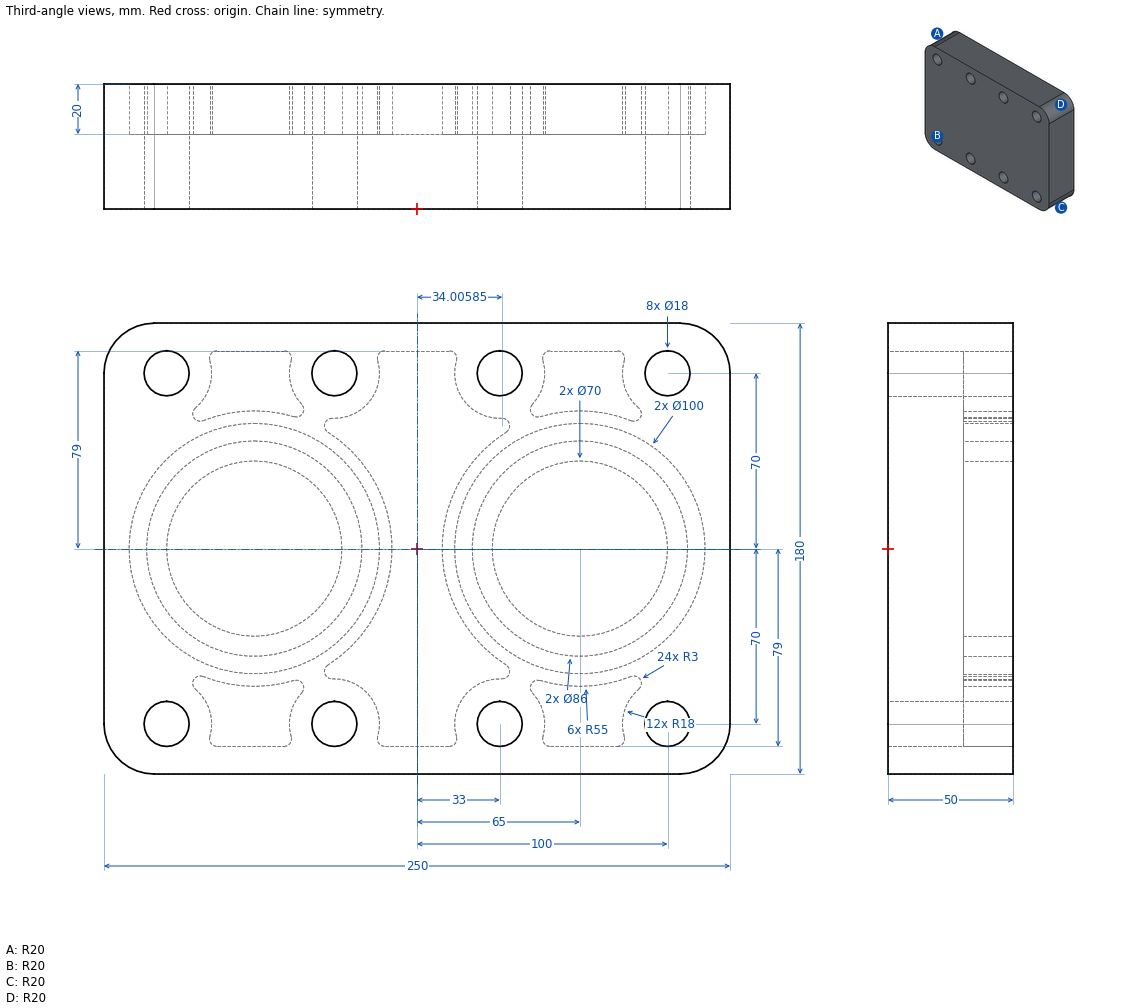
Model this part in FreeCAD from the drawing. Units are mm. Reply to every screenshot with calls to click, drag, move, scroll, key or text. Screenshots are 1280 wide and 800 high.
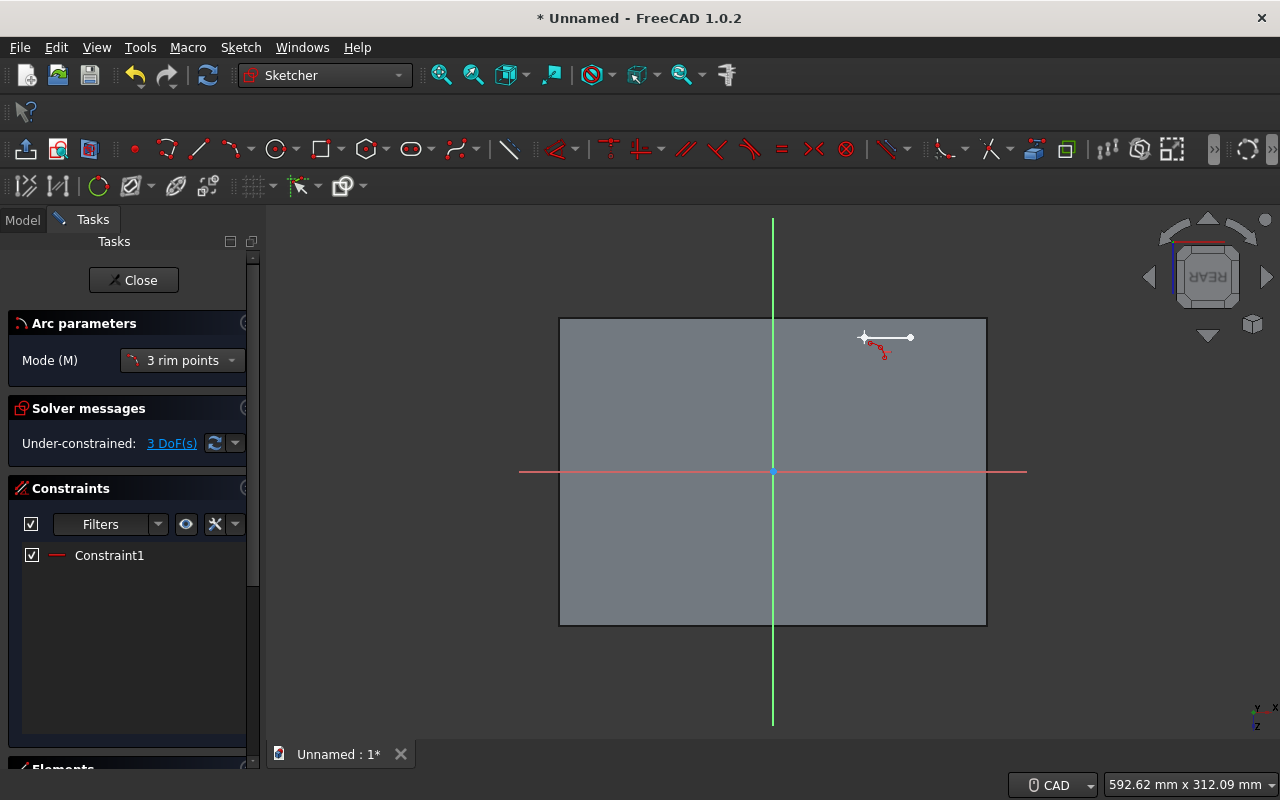
click(864, 338)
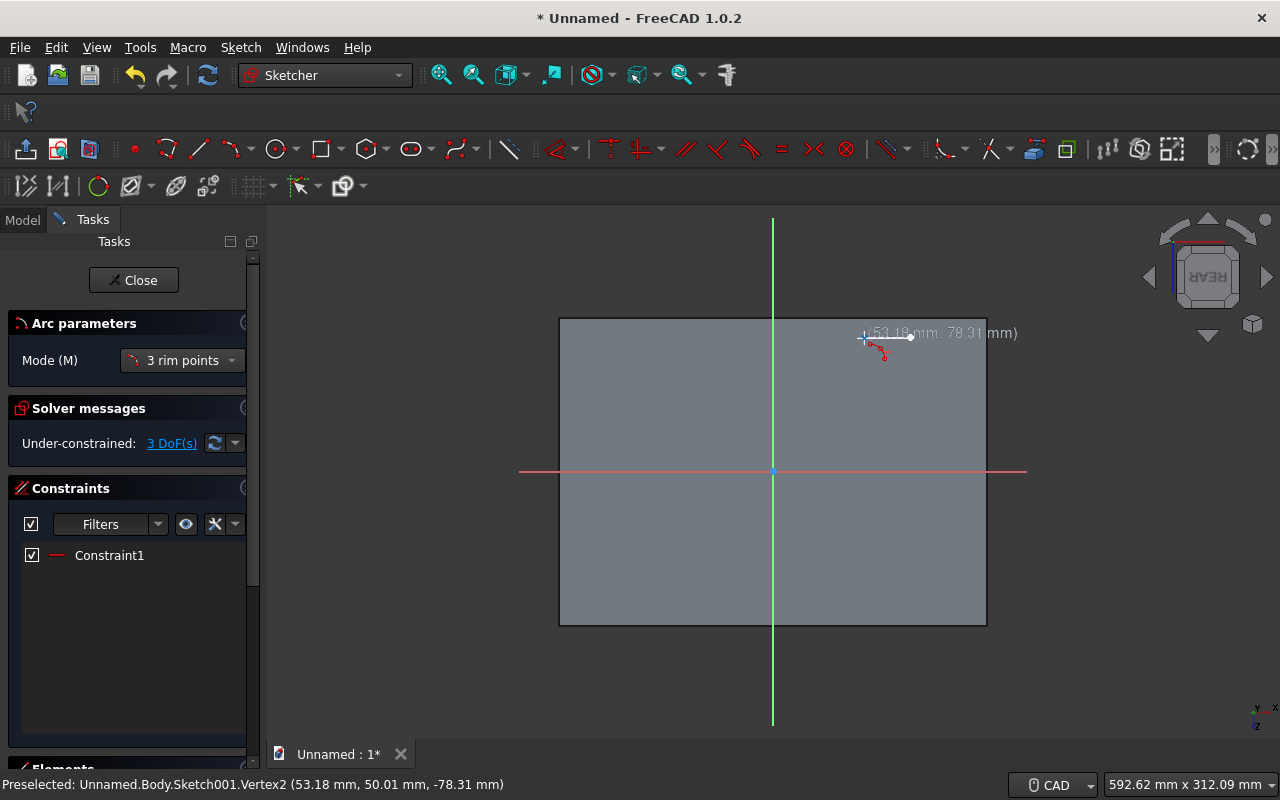
scroll(859, 343, up, 4)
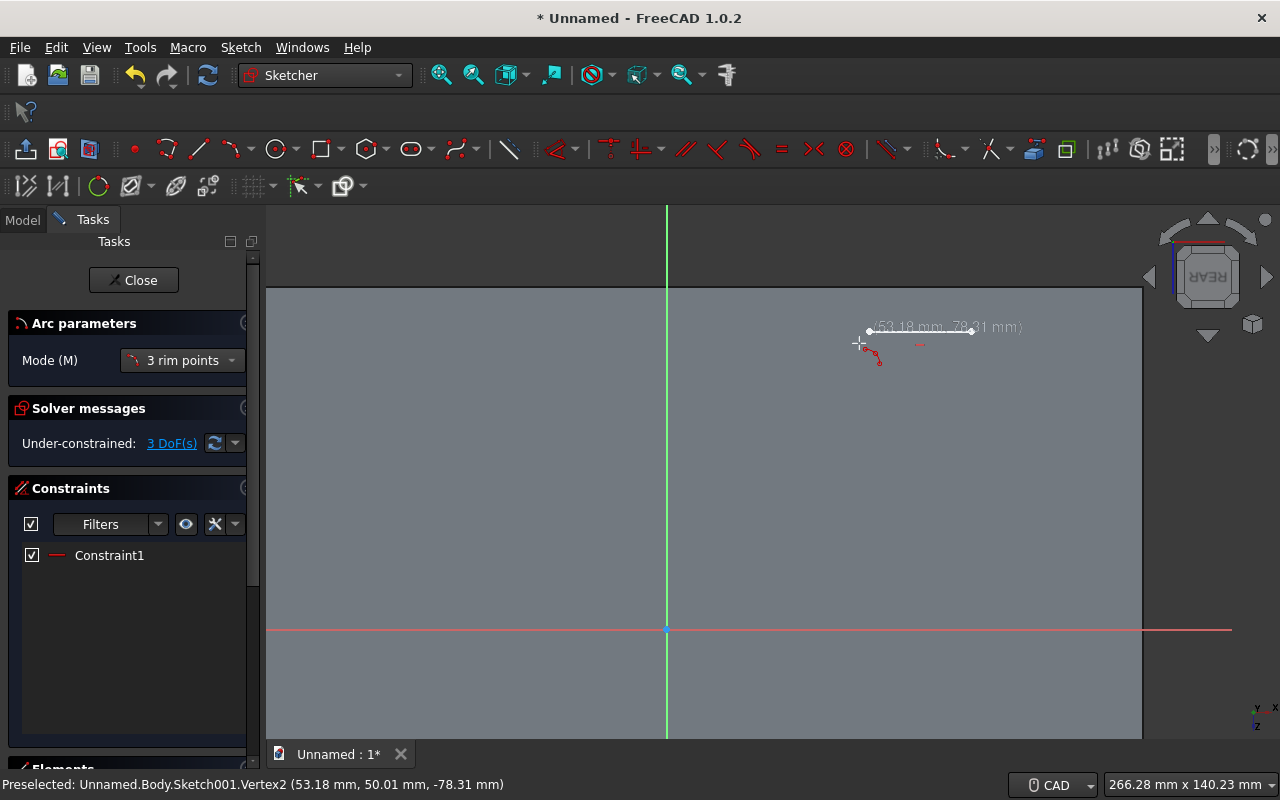
click(858, 344)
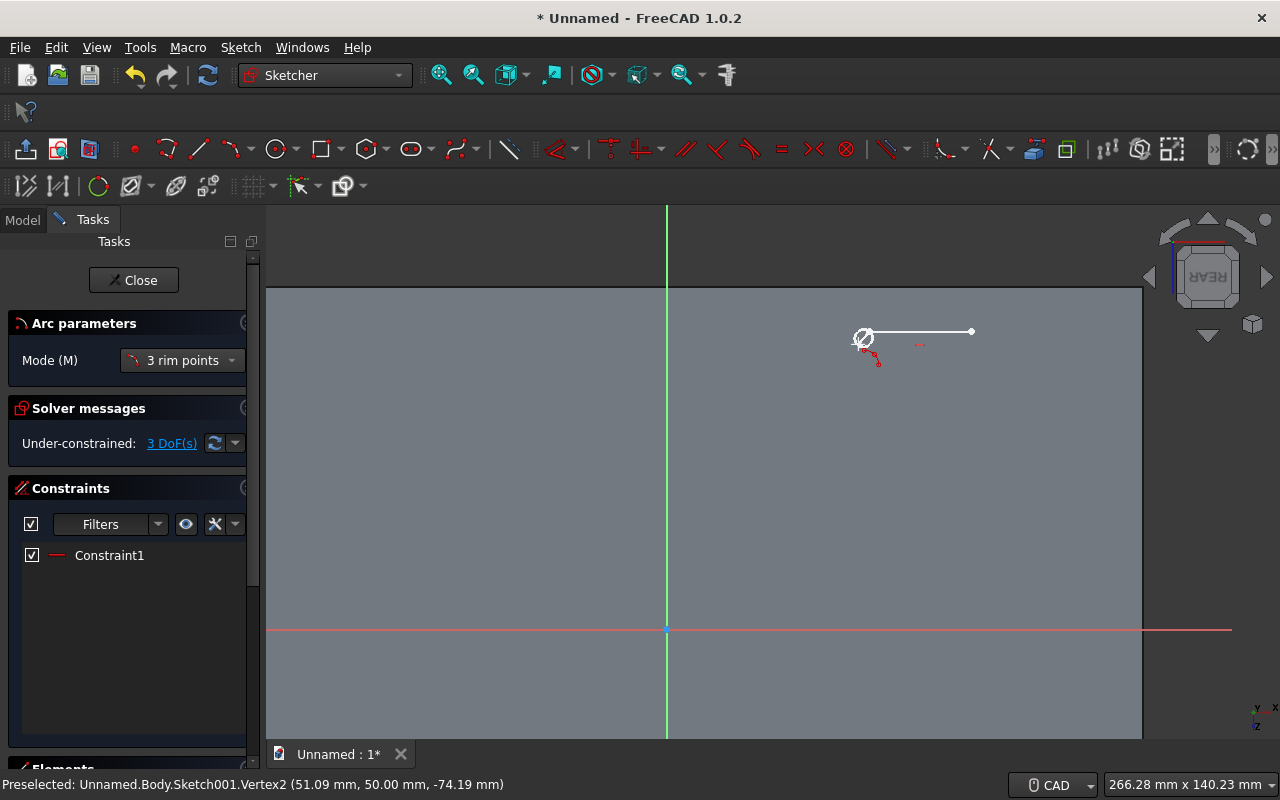
scroll(860, 334, up, 7)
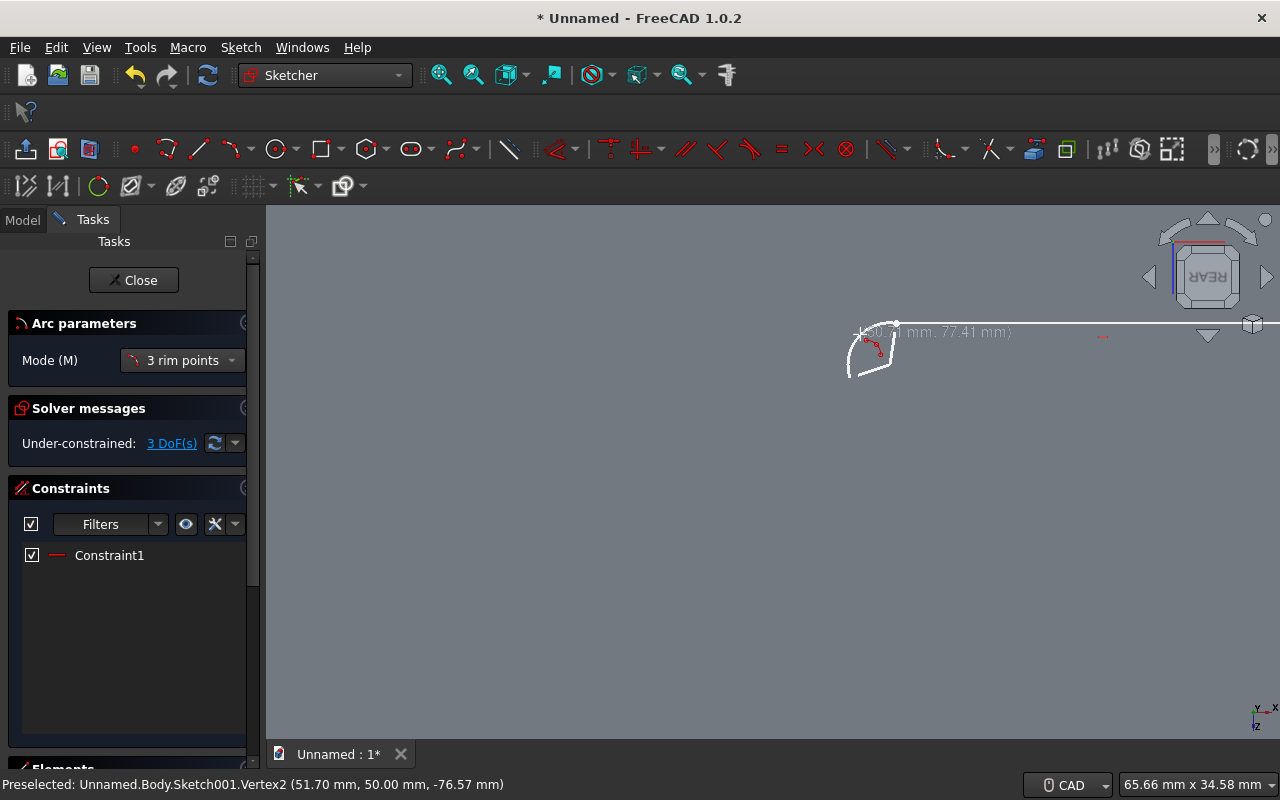
click(858, 331)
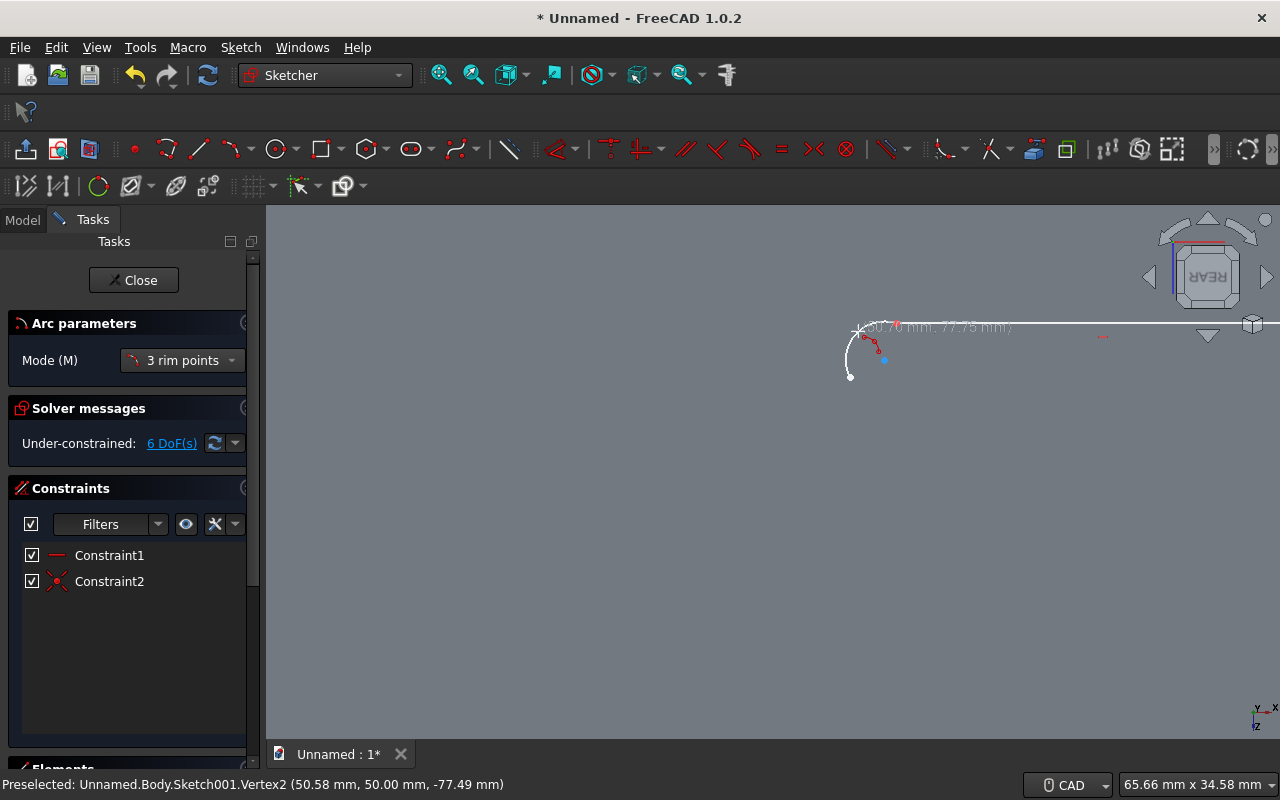
scroll(803, 306, down, 10)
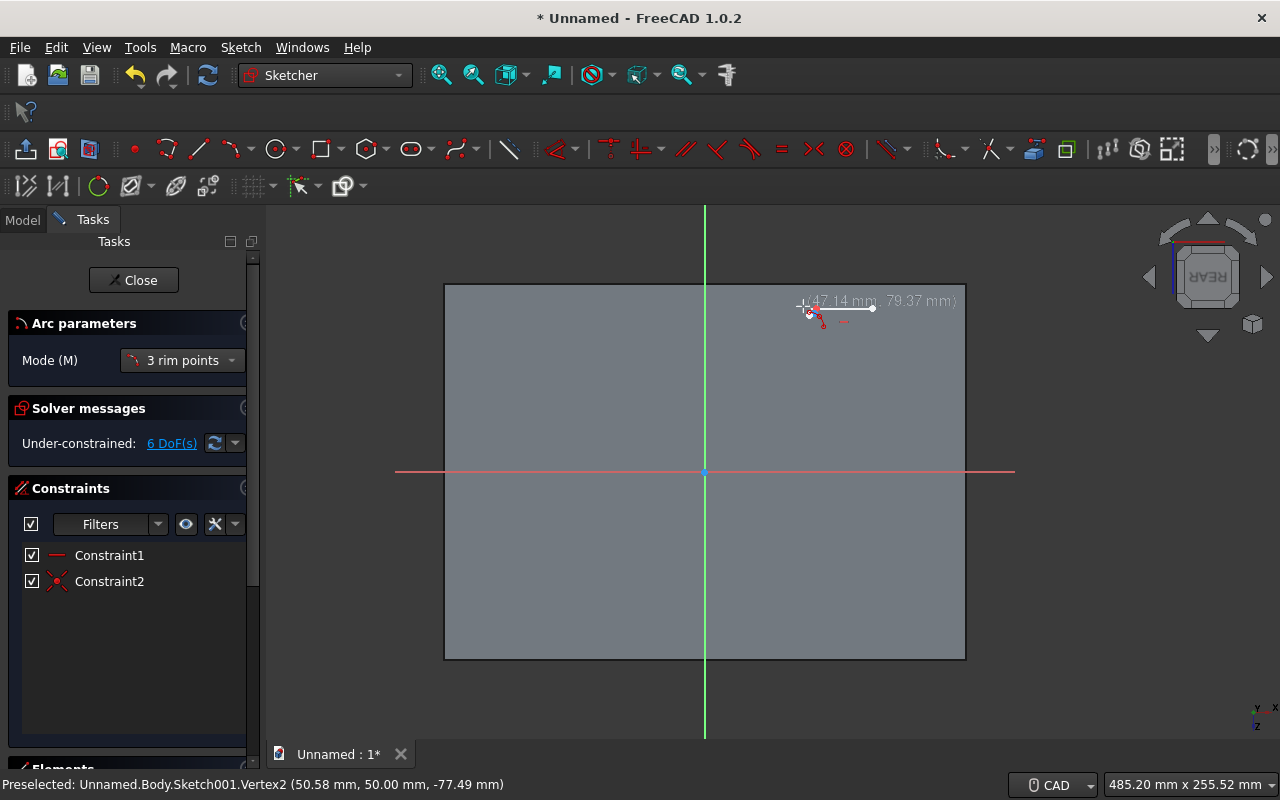
scroll(810, 315, up, 5)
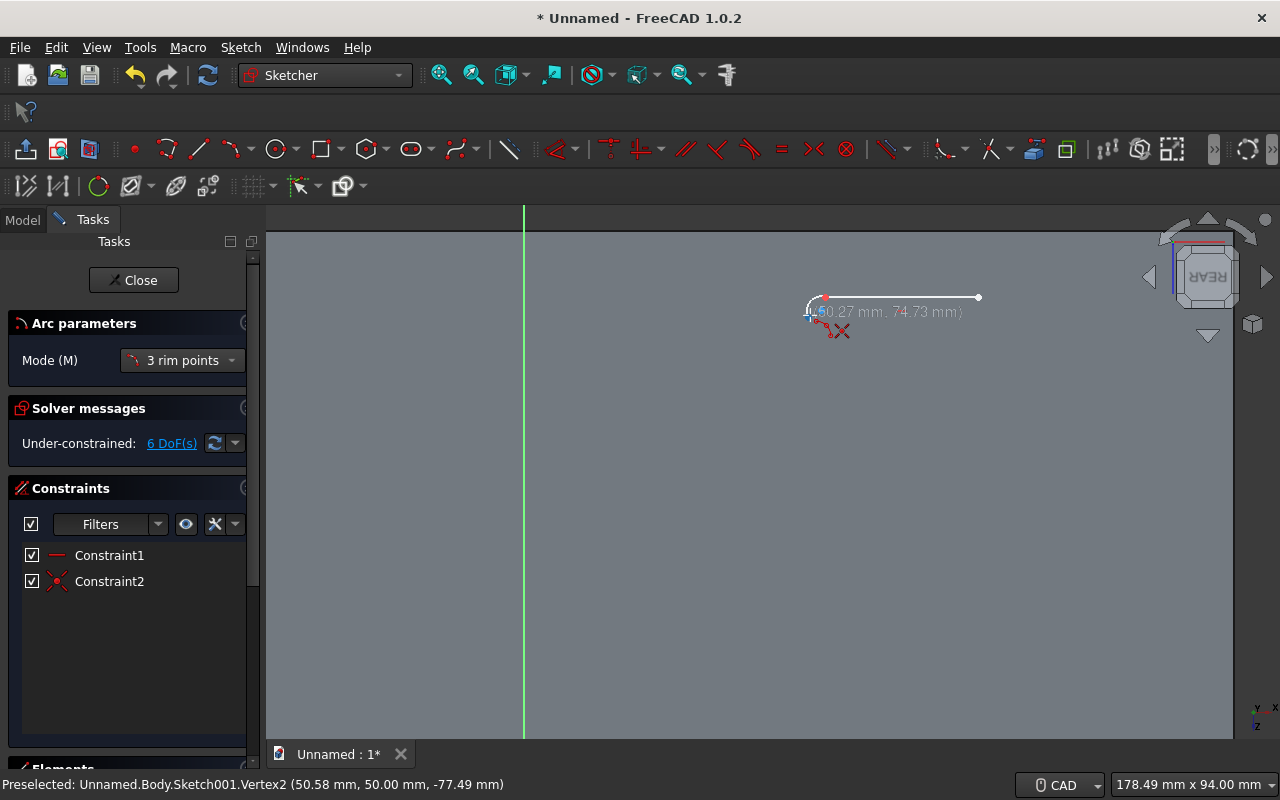
click(809, 317)
click(785, 415)
click(810, 368)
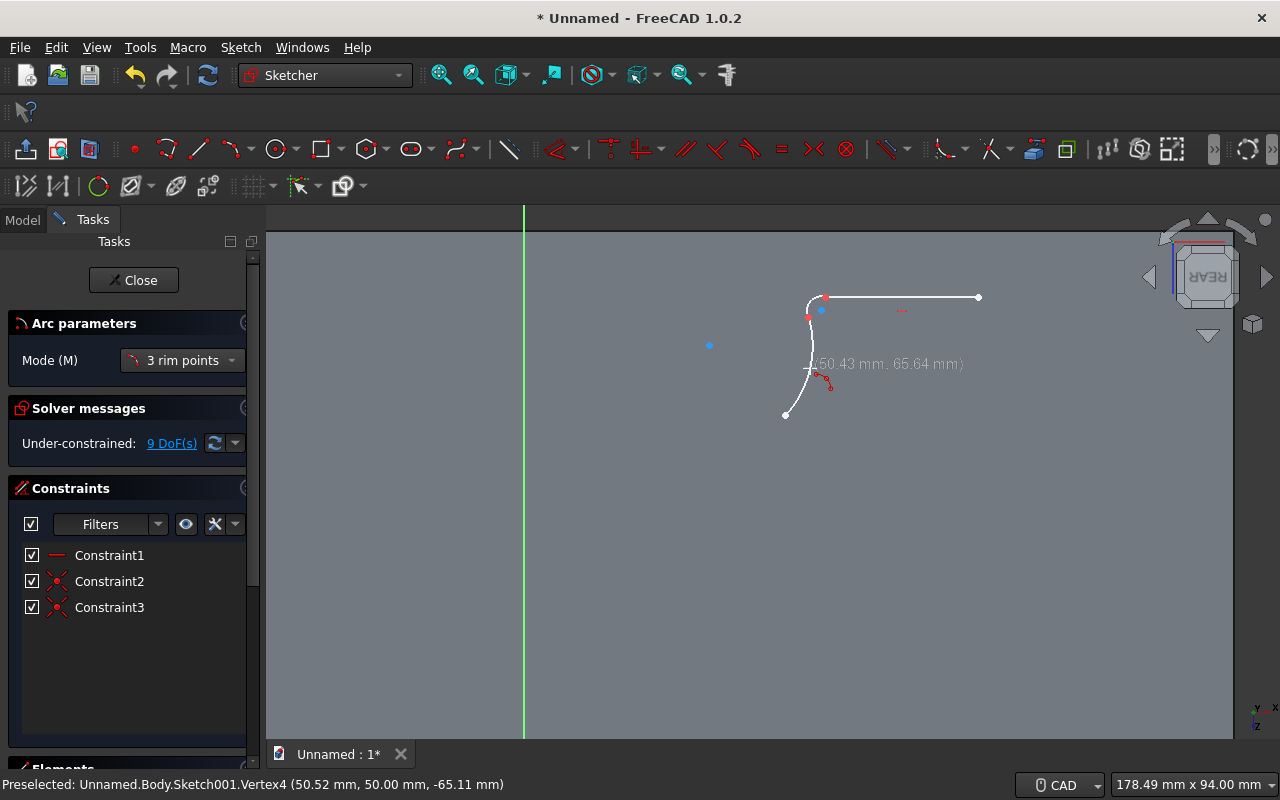
click(785, 416)
click(802, 443)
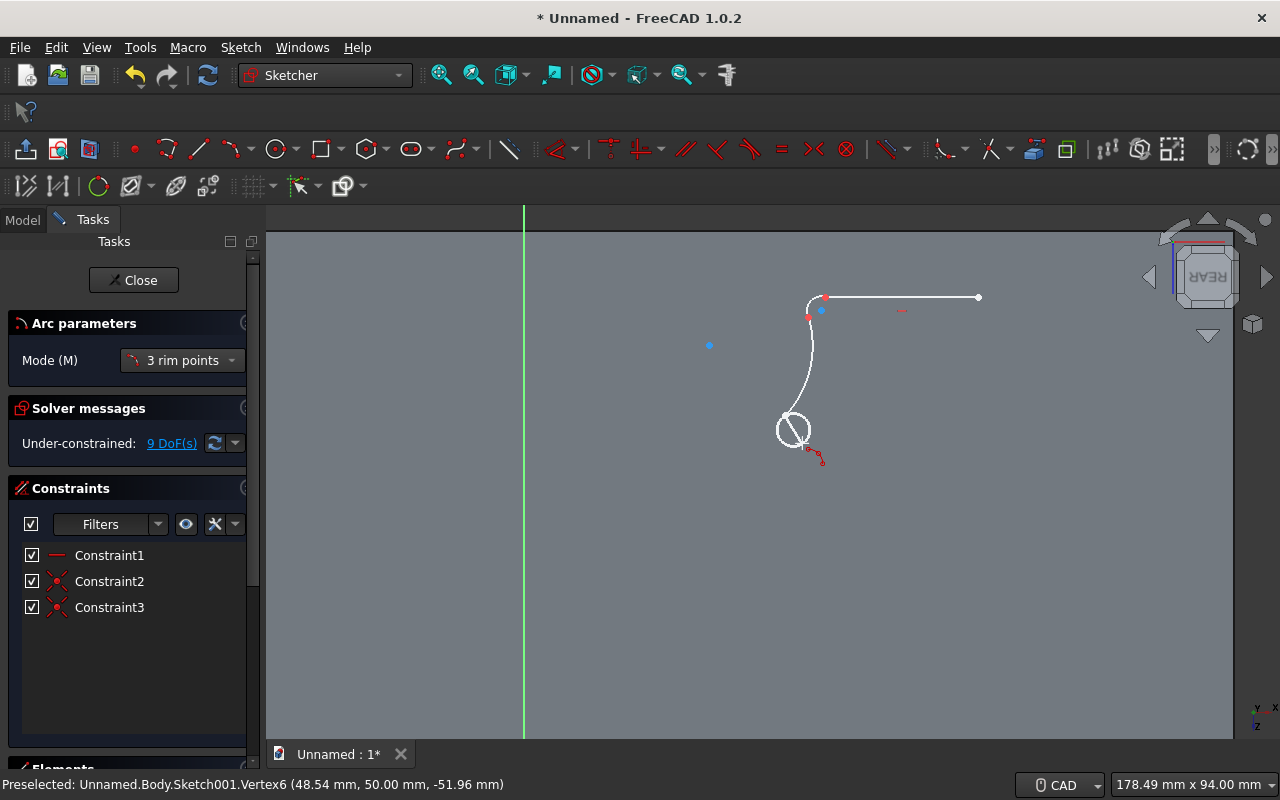
scroll(783, 435, up, 2)